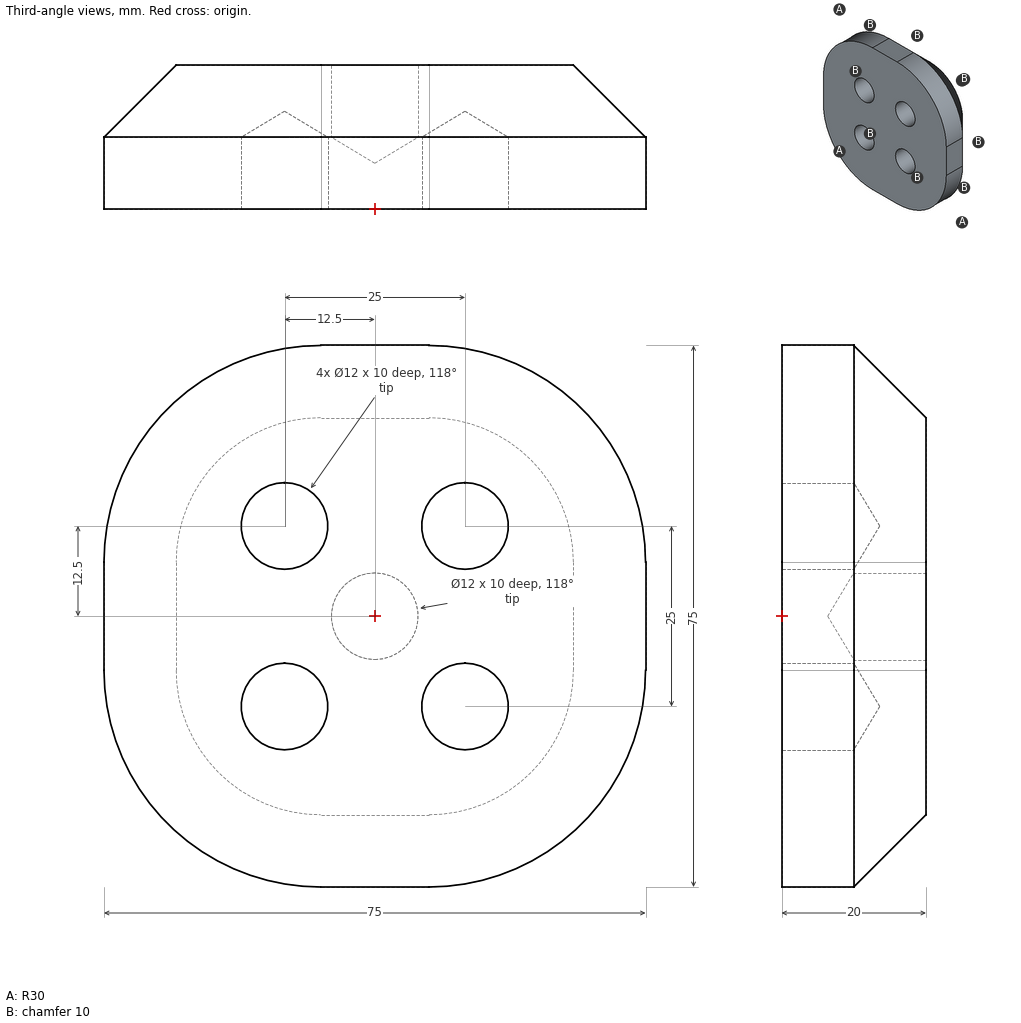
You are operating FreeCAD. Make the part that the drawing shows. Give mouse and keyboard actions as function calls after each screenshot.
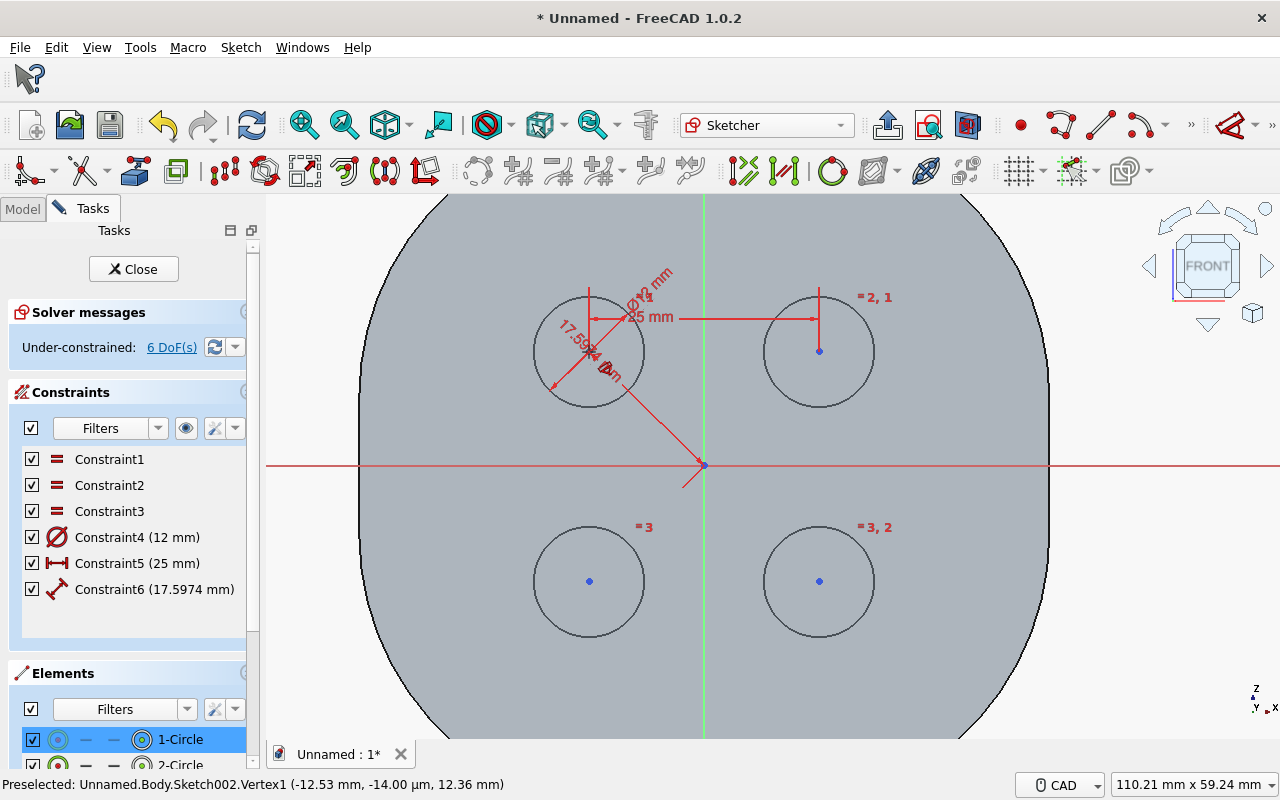
click(819, 582)
click(651, 616)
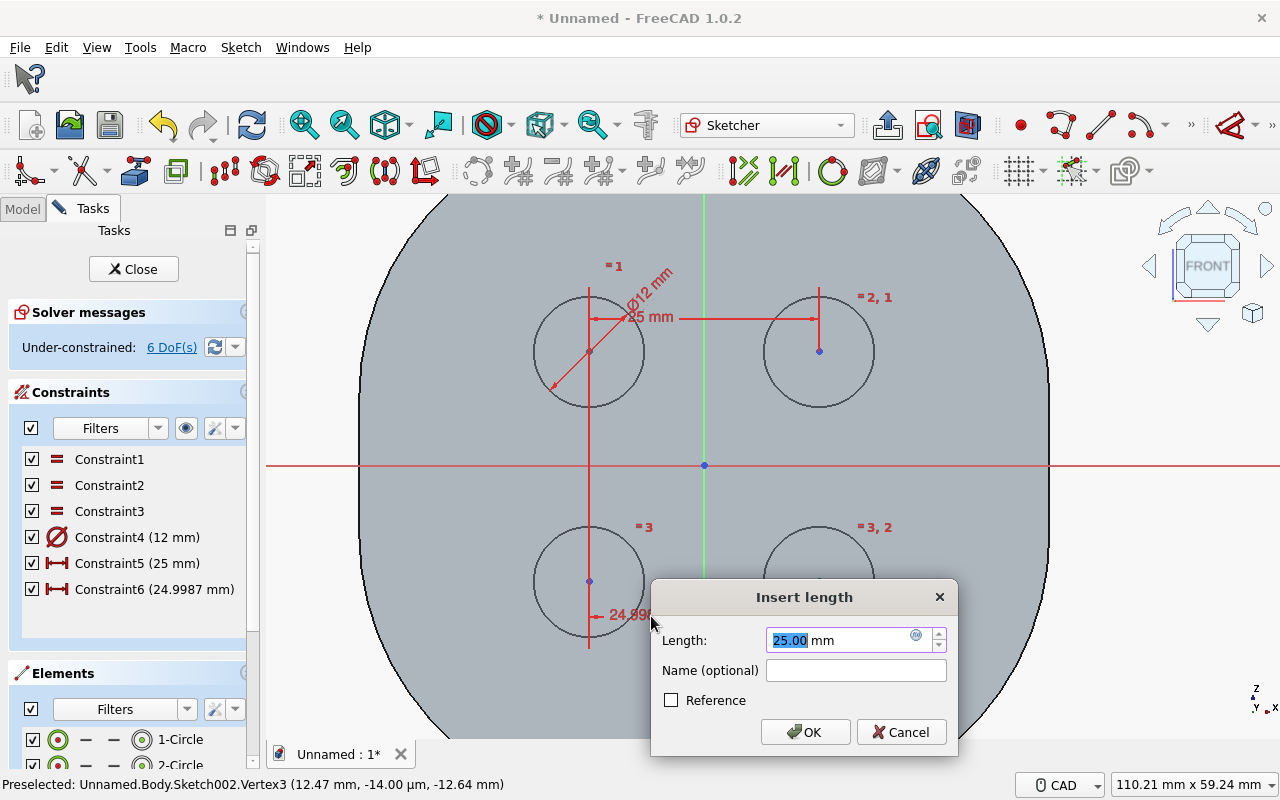
text(25)
key(Return)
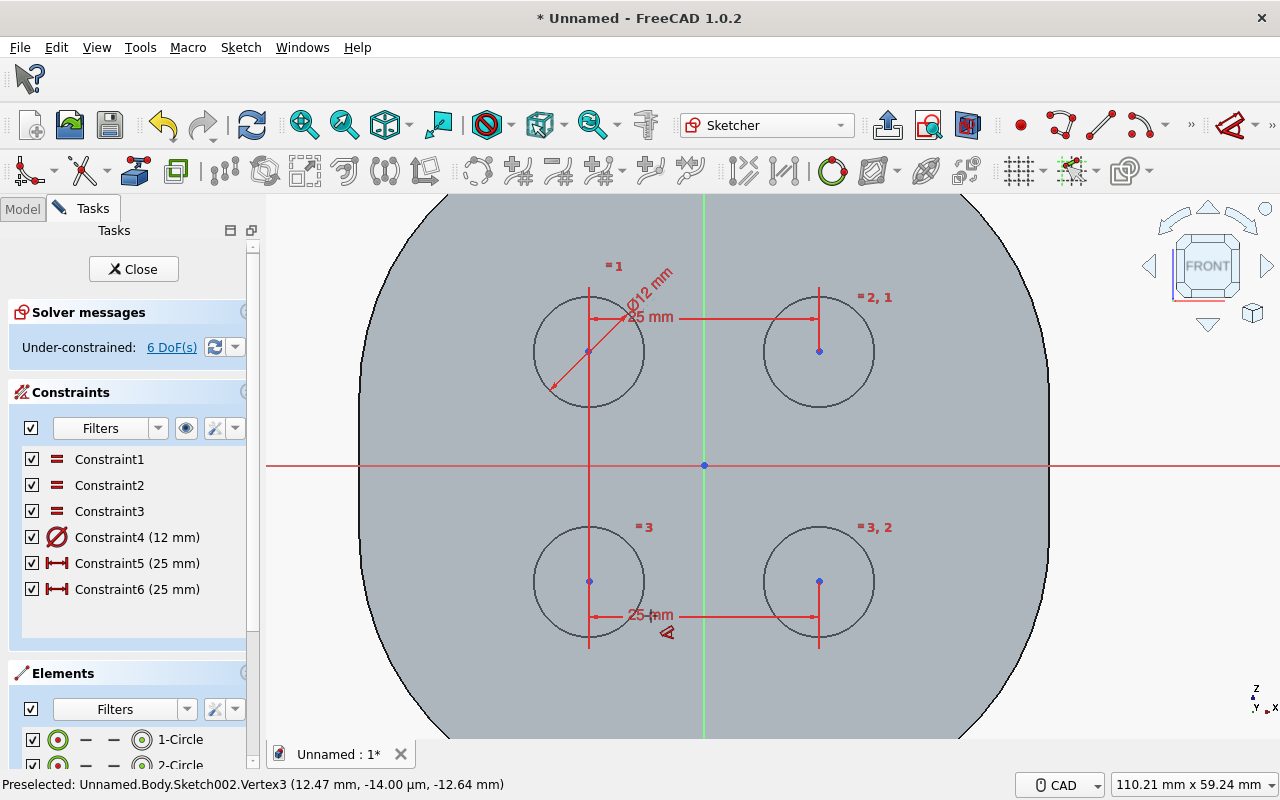
click(819, 352)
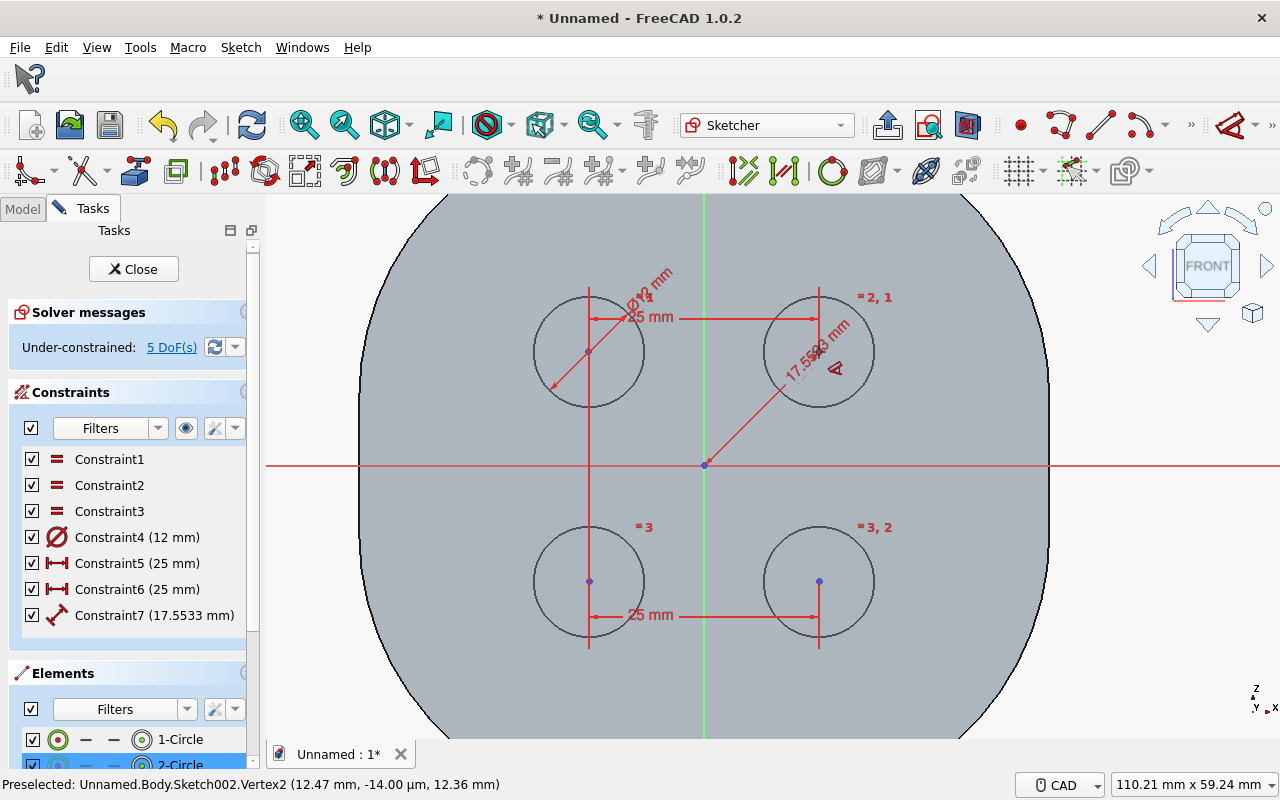
click(819, 582)
click(853, 414)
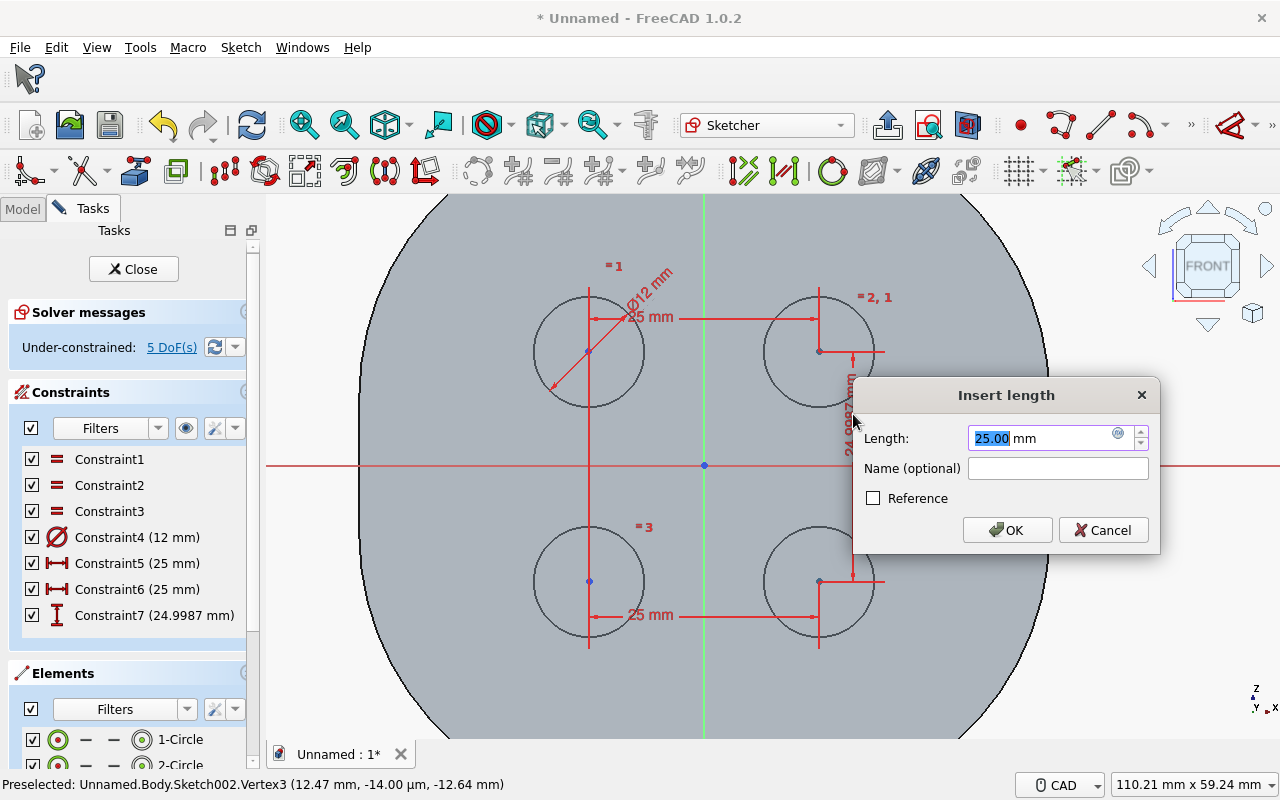
text(25)
key(Return)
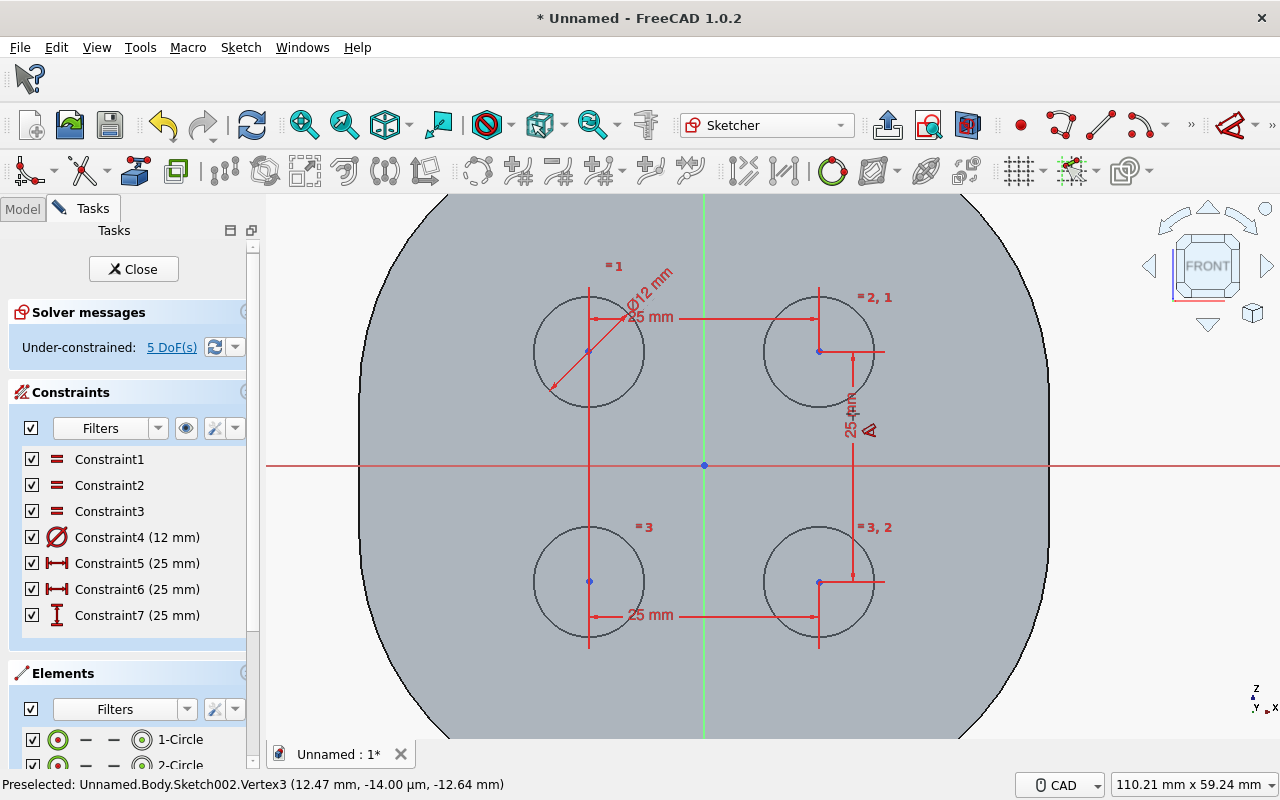
click(589, 352)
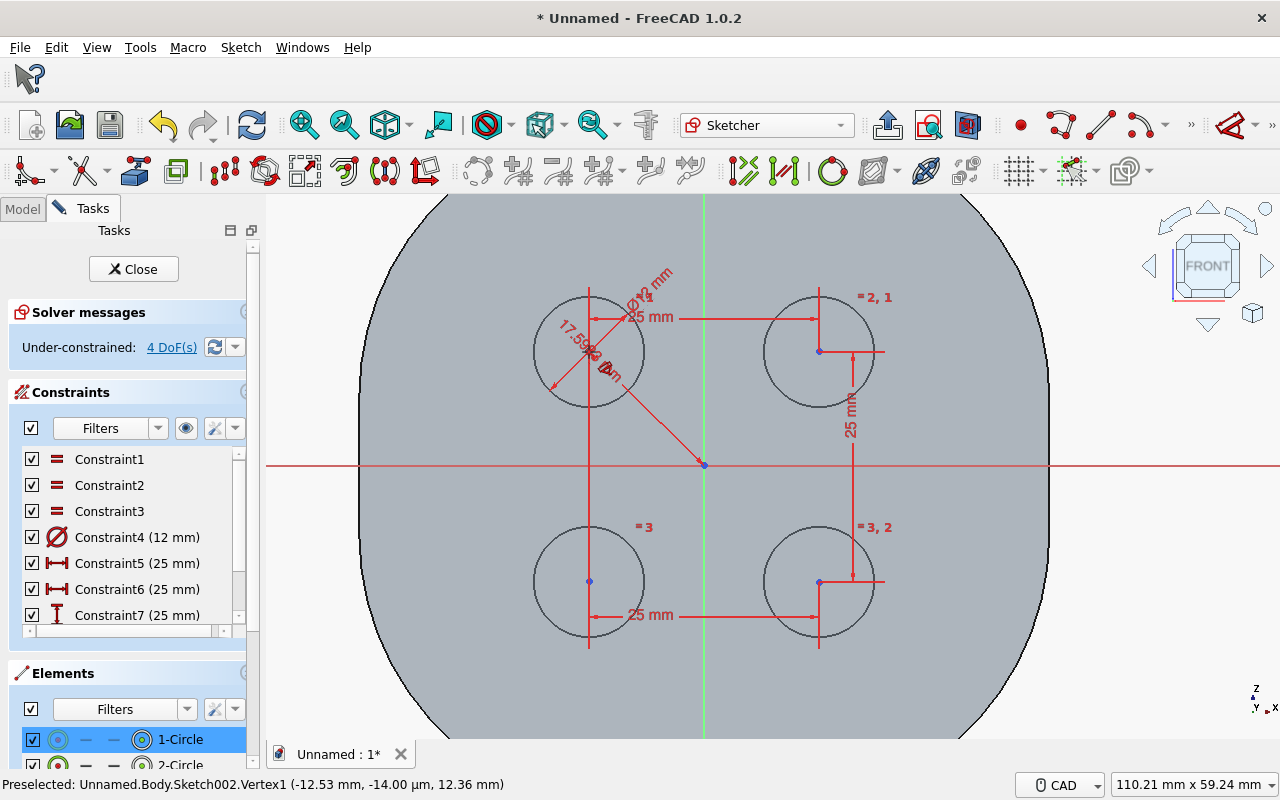
click(819, 582)
click(555, 414)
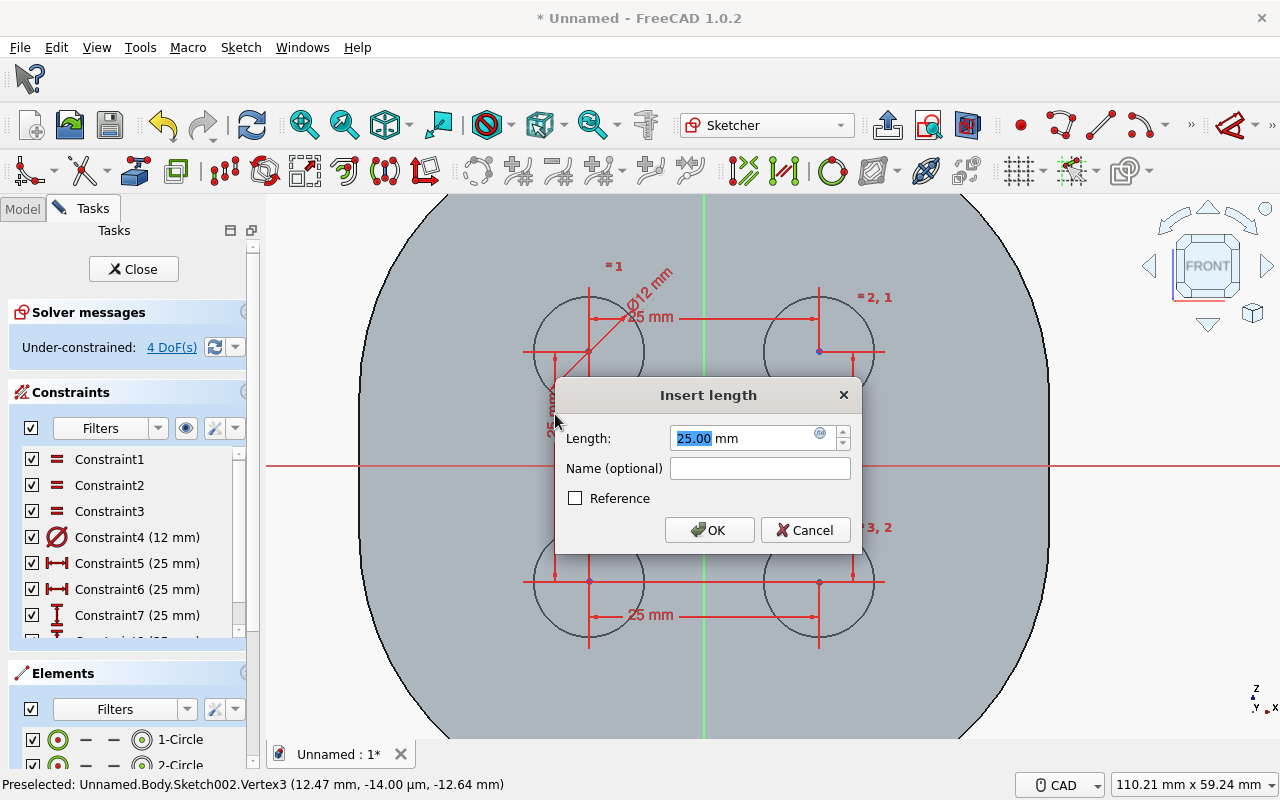
text(25)
key(Return)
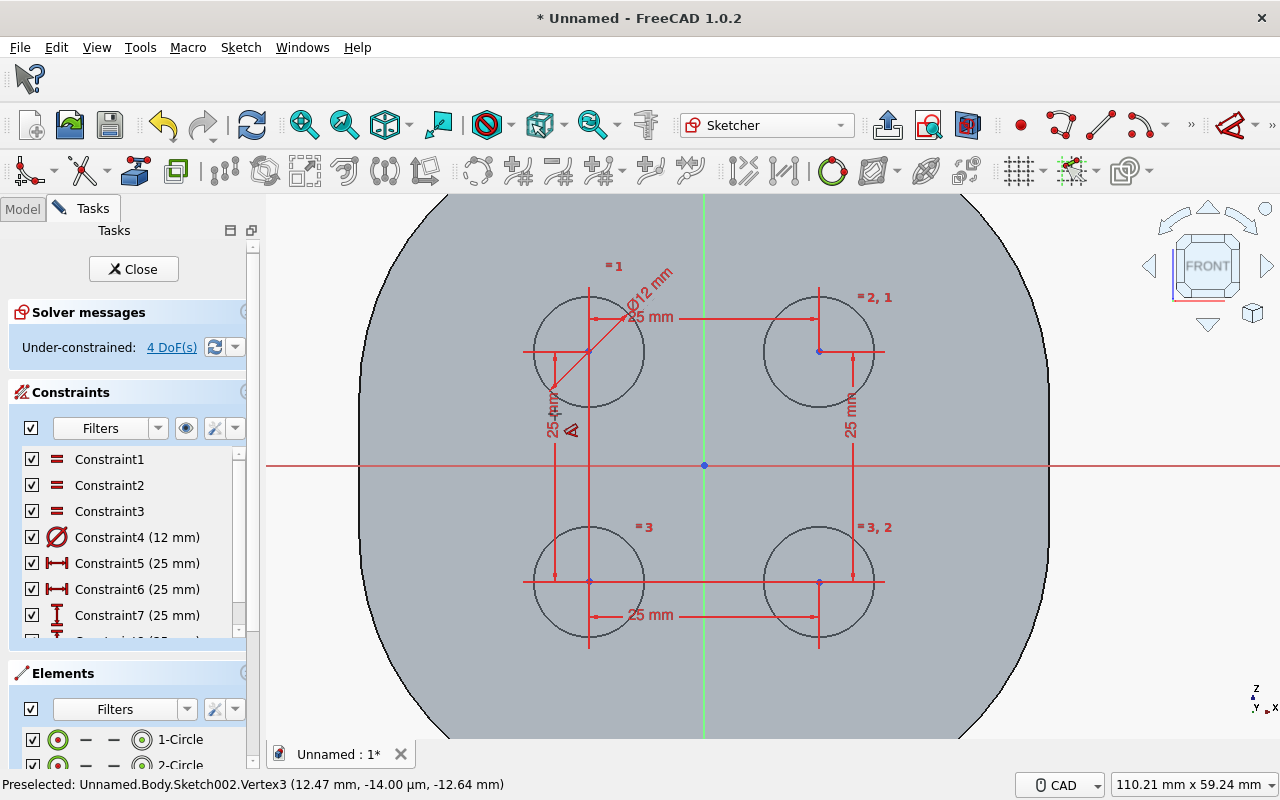
click(819, 582)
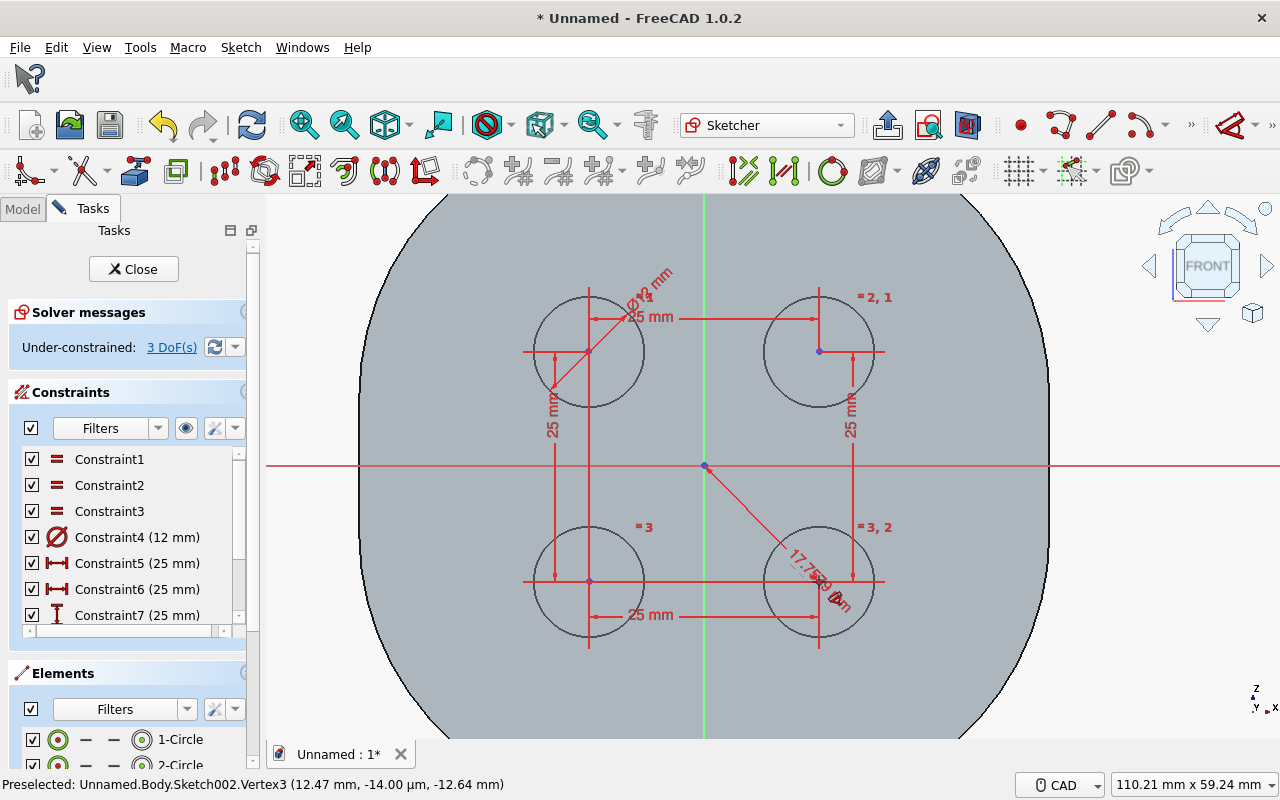
click(589, 582)
click(757, 616)